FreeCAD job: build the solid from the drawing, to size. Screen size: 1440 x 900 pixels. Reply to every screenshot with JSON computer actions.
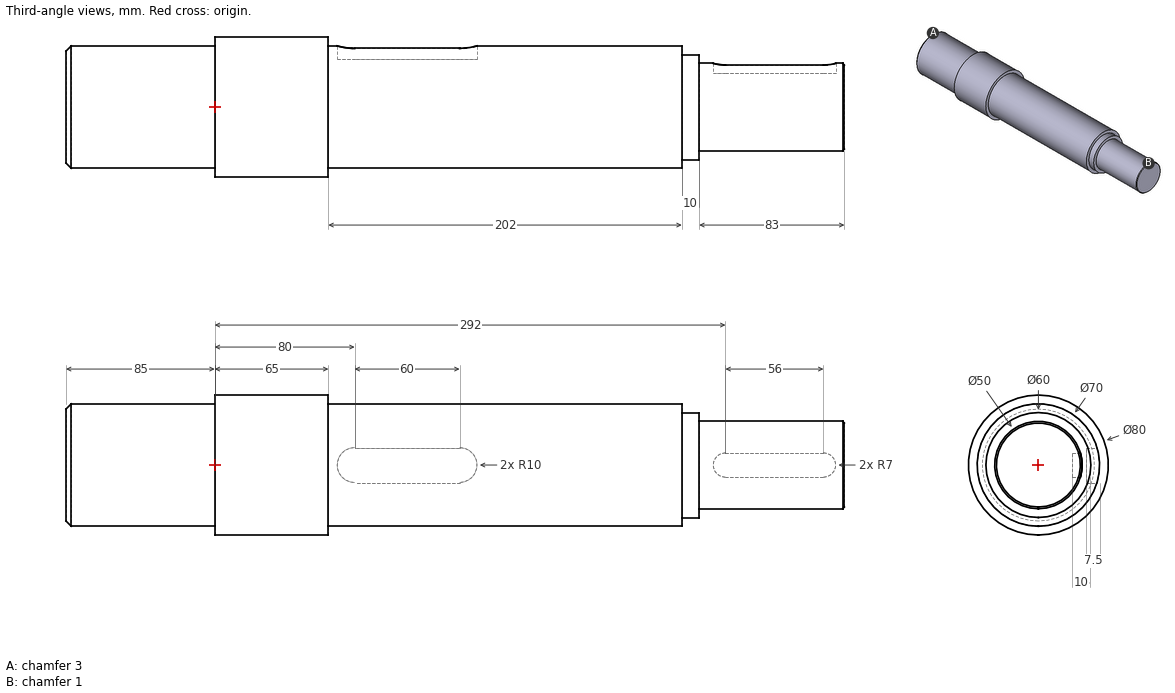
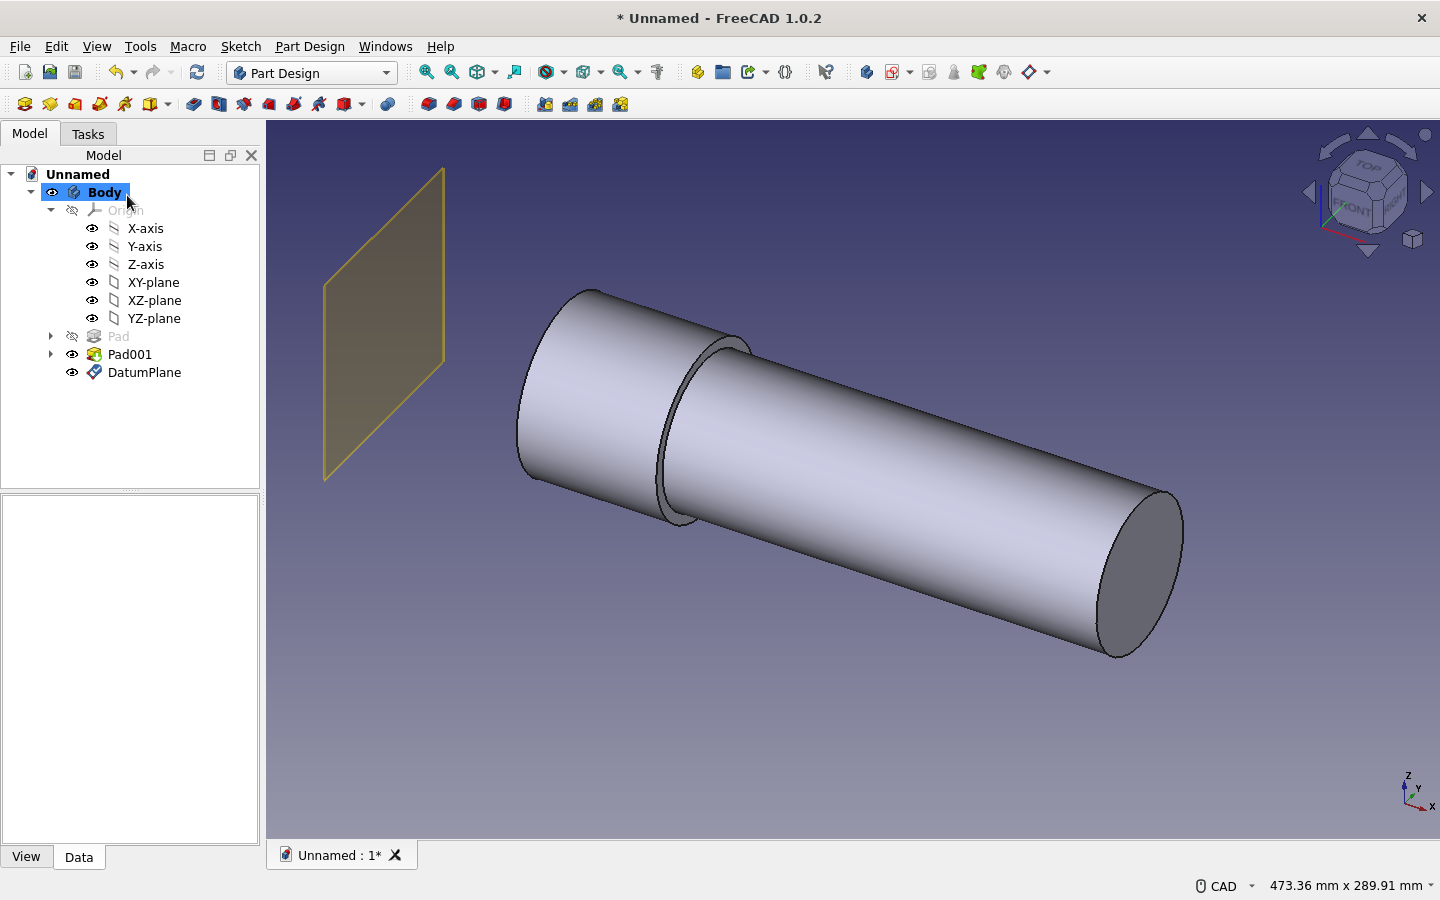
{"action": "left_click", "coordinate": [117, 372]}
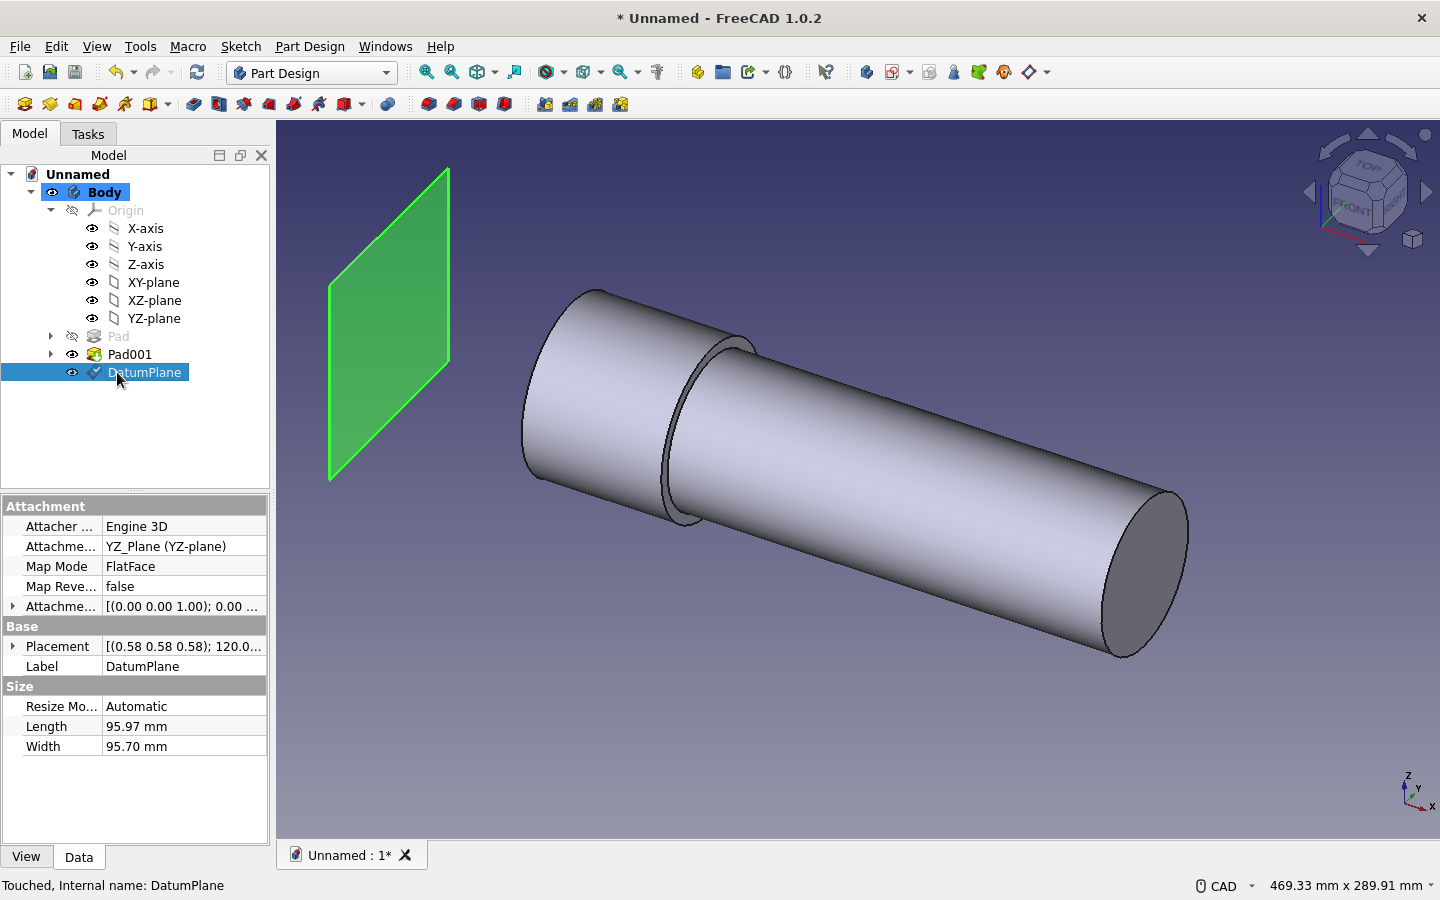
{"action": "left_click", "coordinate": [892, 72]}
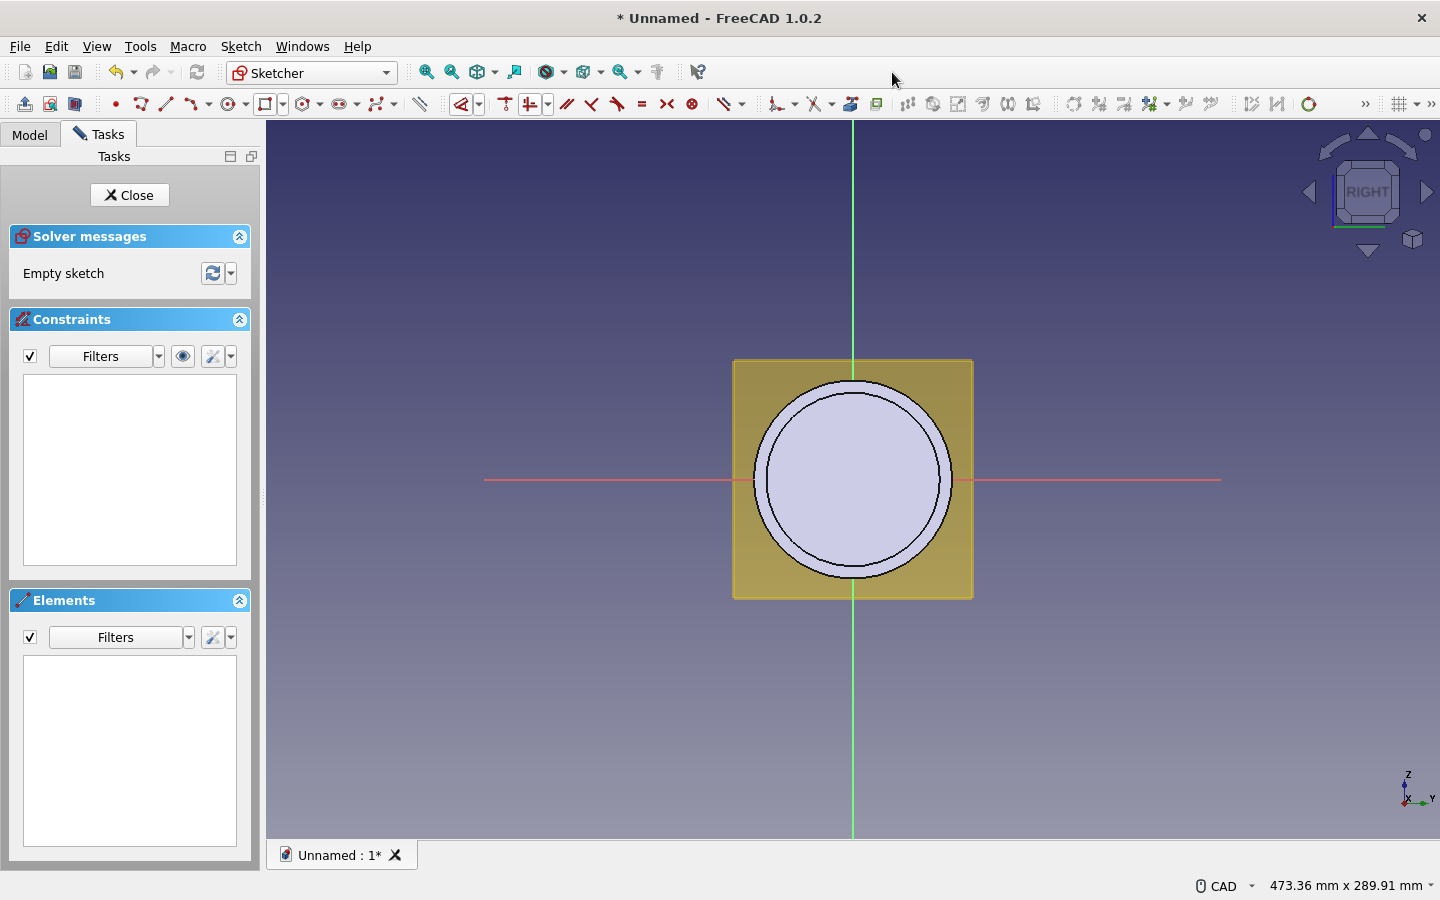
{"action": "key", "text": "q s"}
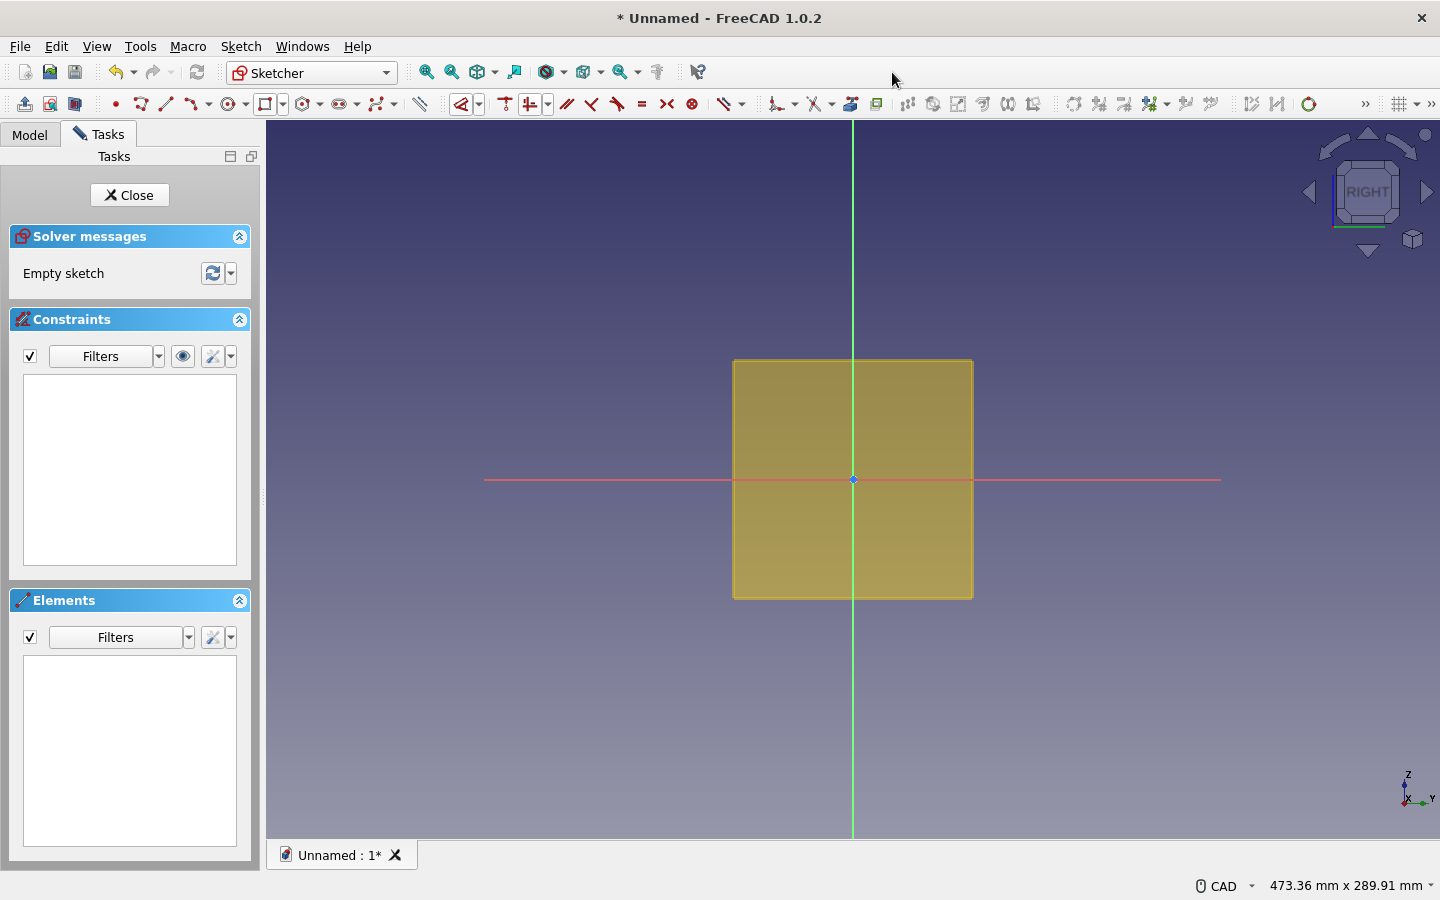
{"action": "scroll", "coordinate": [893, 480], "scroll_direction": "up", "scroll_amount": 5}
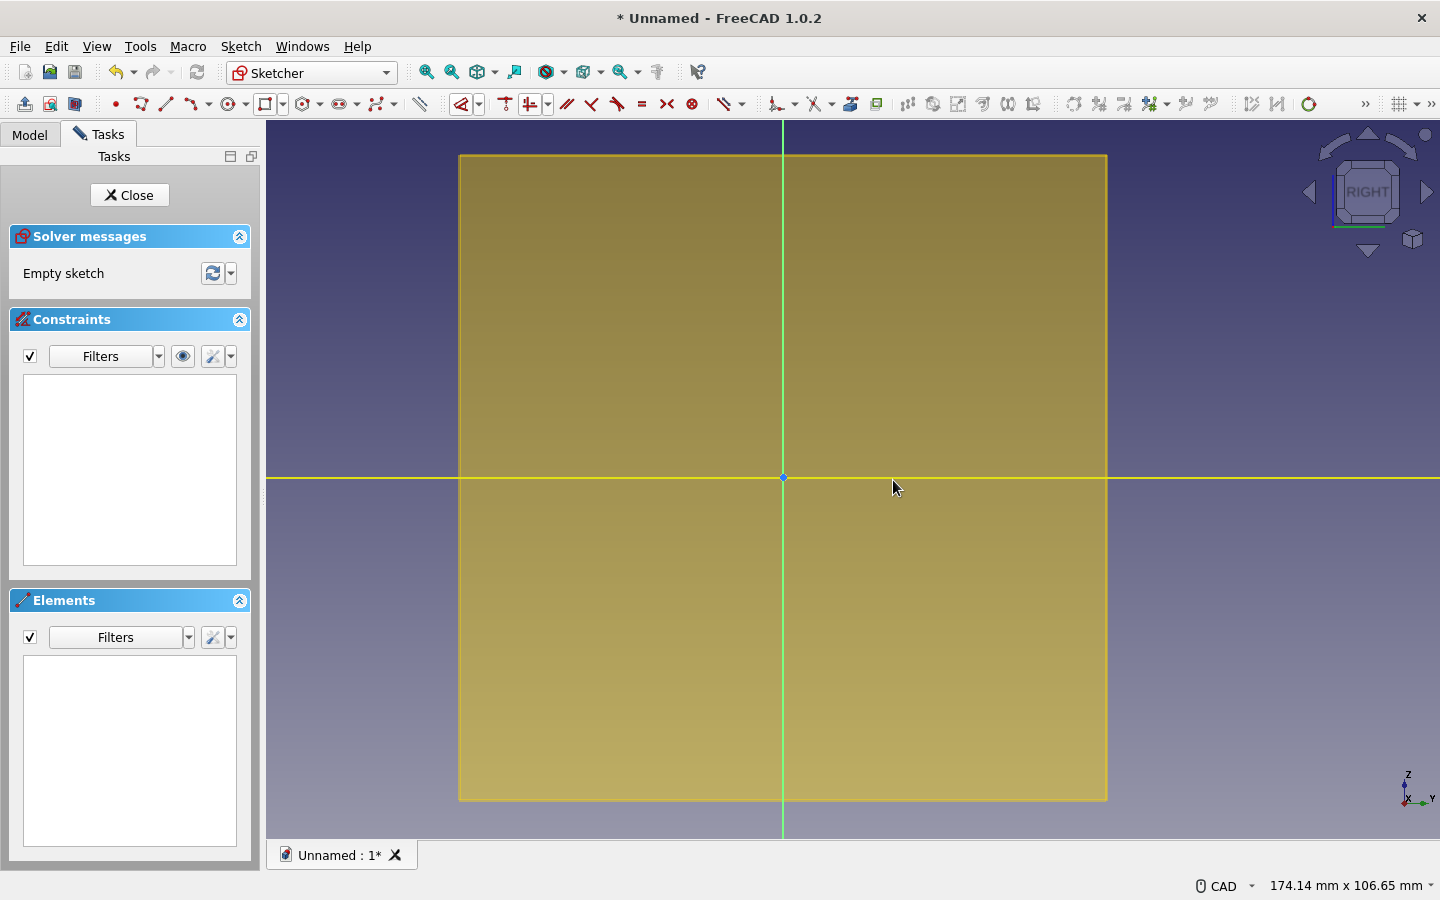
{"action": "left_click", "coordinate": [228, 104]}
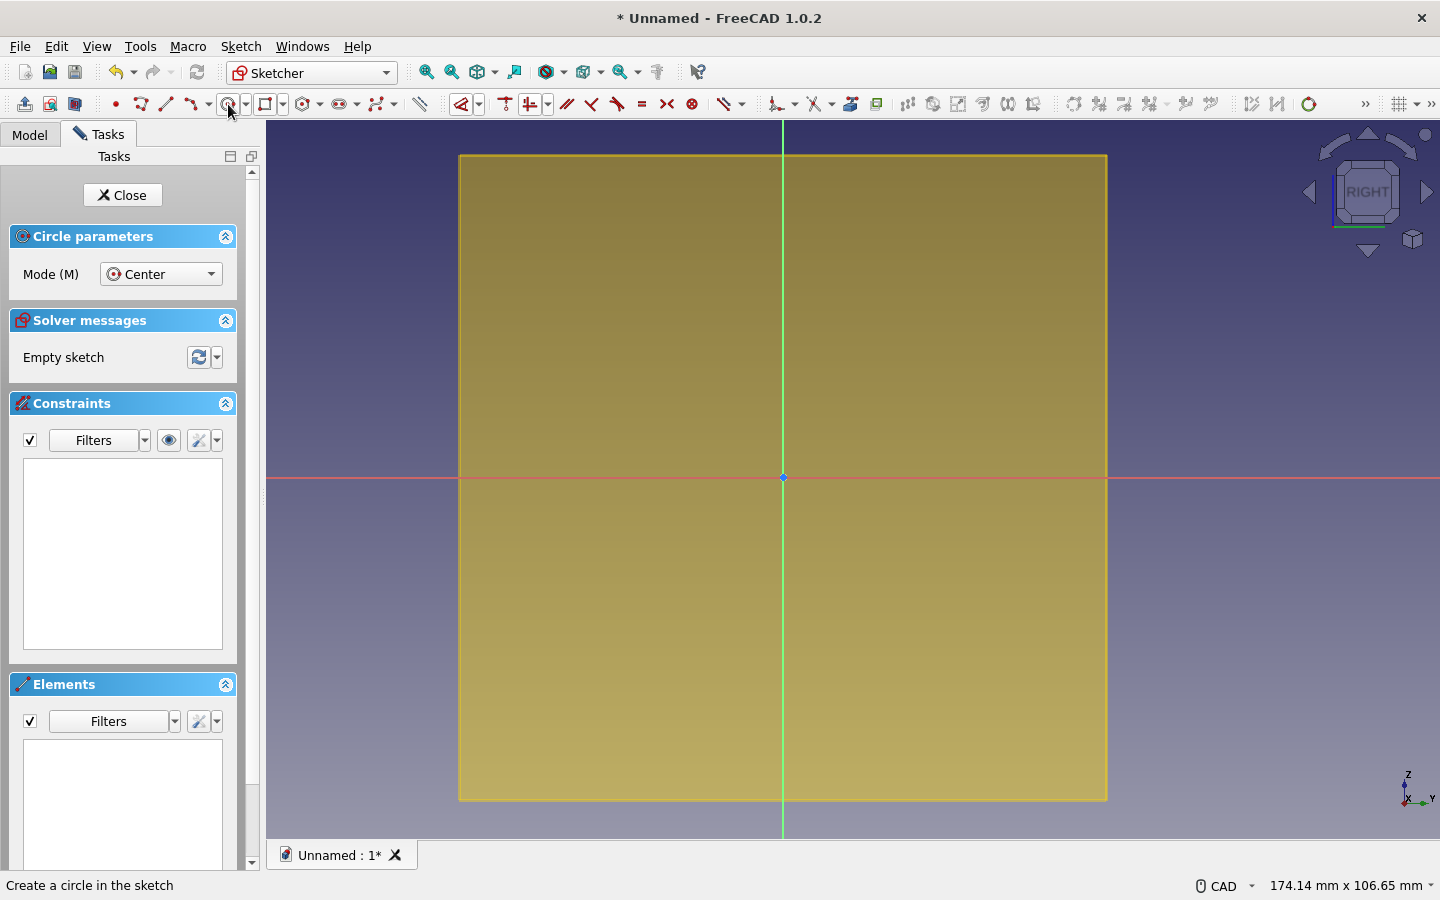
{"action": "left_click", "coordinate": [783, 478]}
{"action": "left_click", "coordinate": [950, 311]}
{"action": "key", "text": "Escape"}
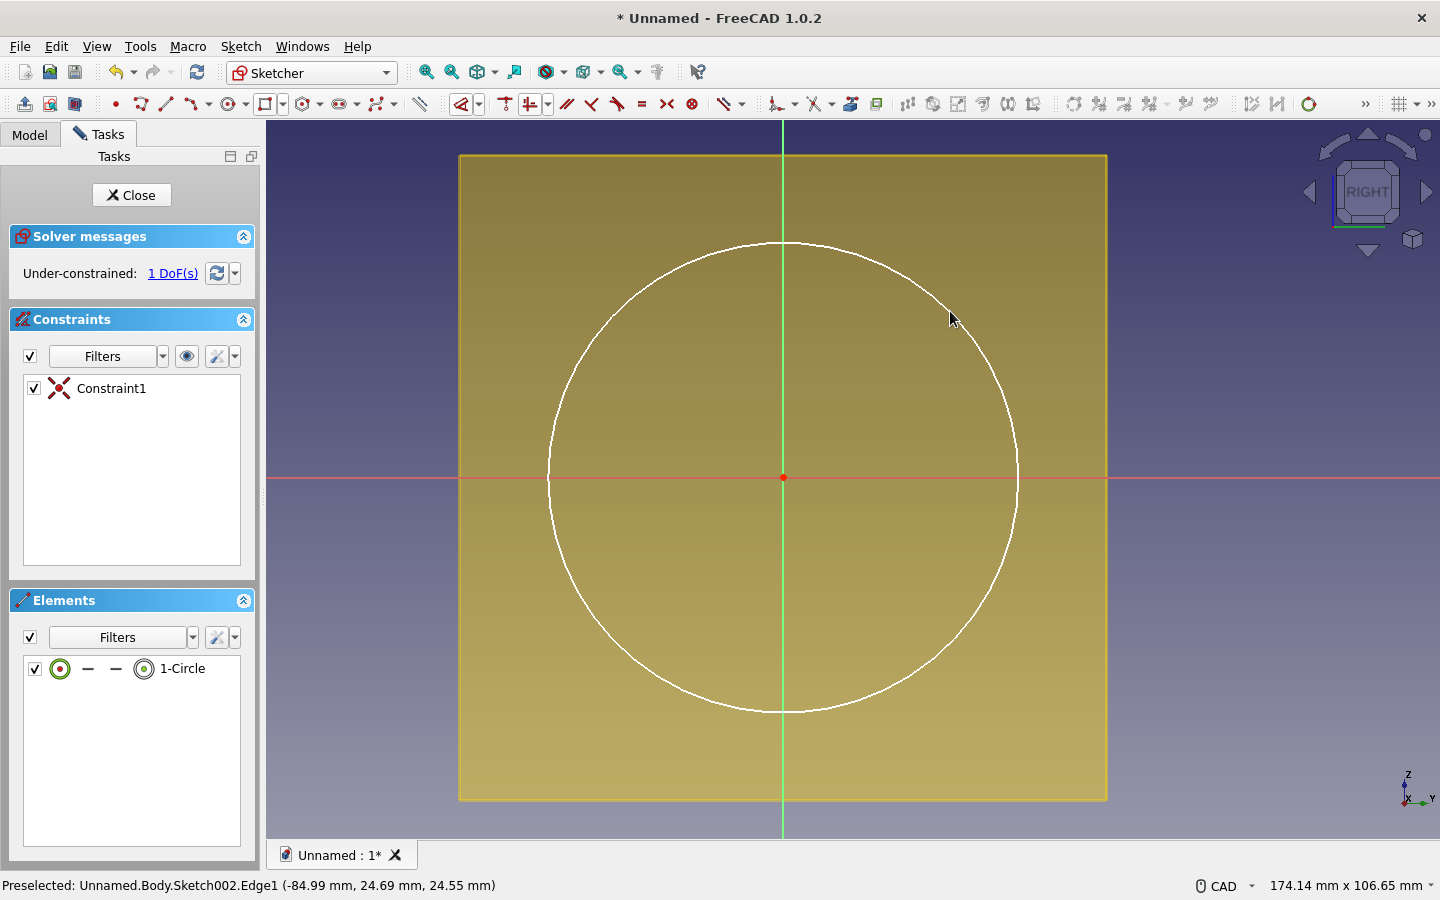
{"action": "key", "text": "d"}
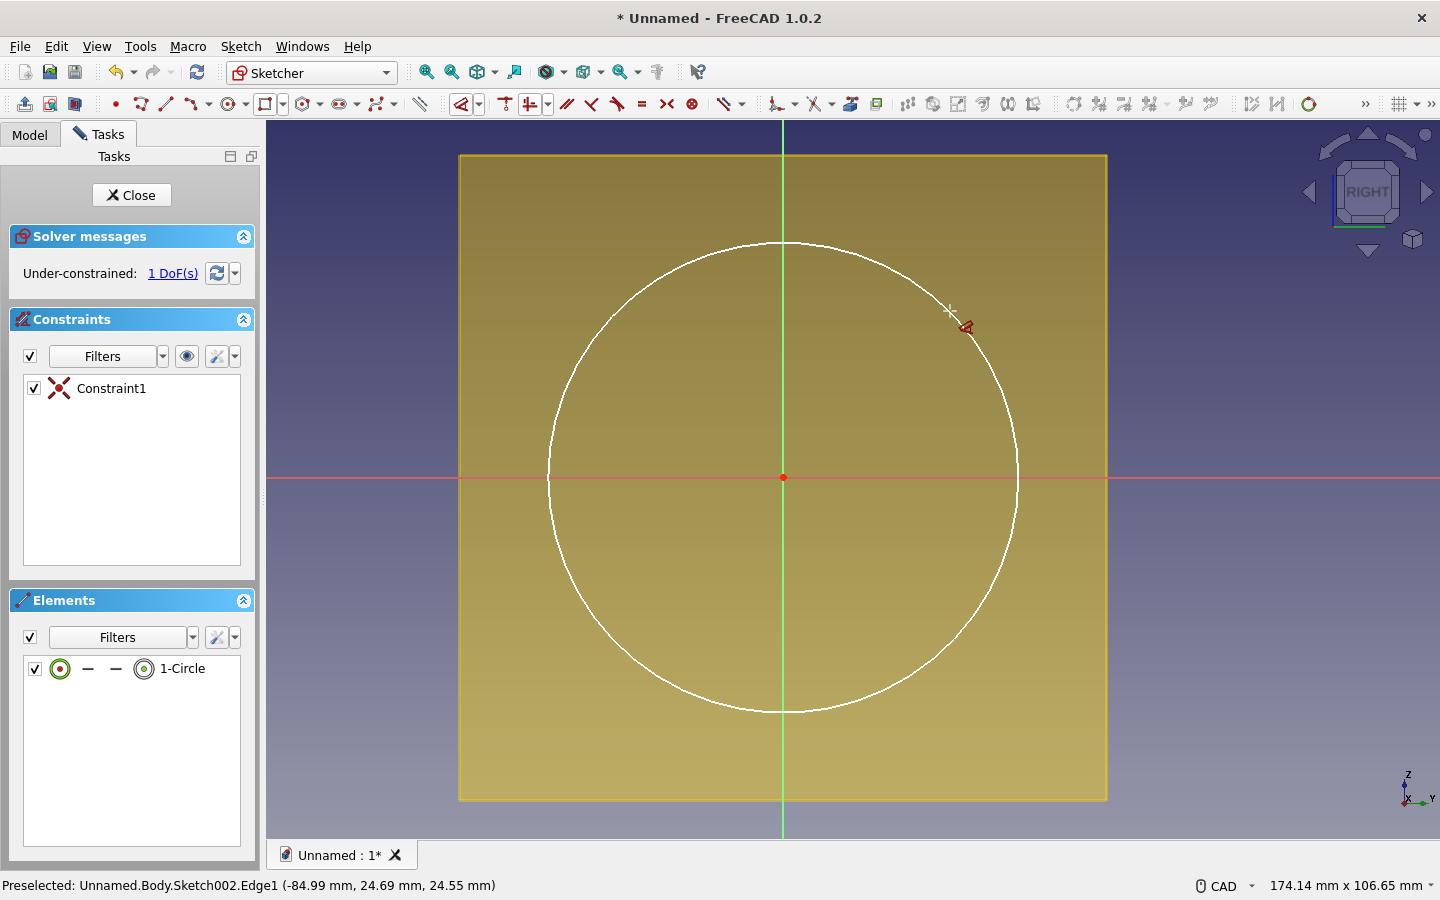
{"action": "left_click", "coordinate": [949, 311]}
{"action": "left_click", "coordinate": [972, 288]}